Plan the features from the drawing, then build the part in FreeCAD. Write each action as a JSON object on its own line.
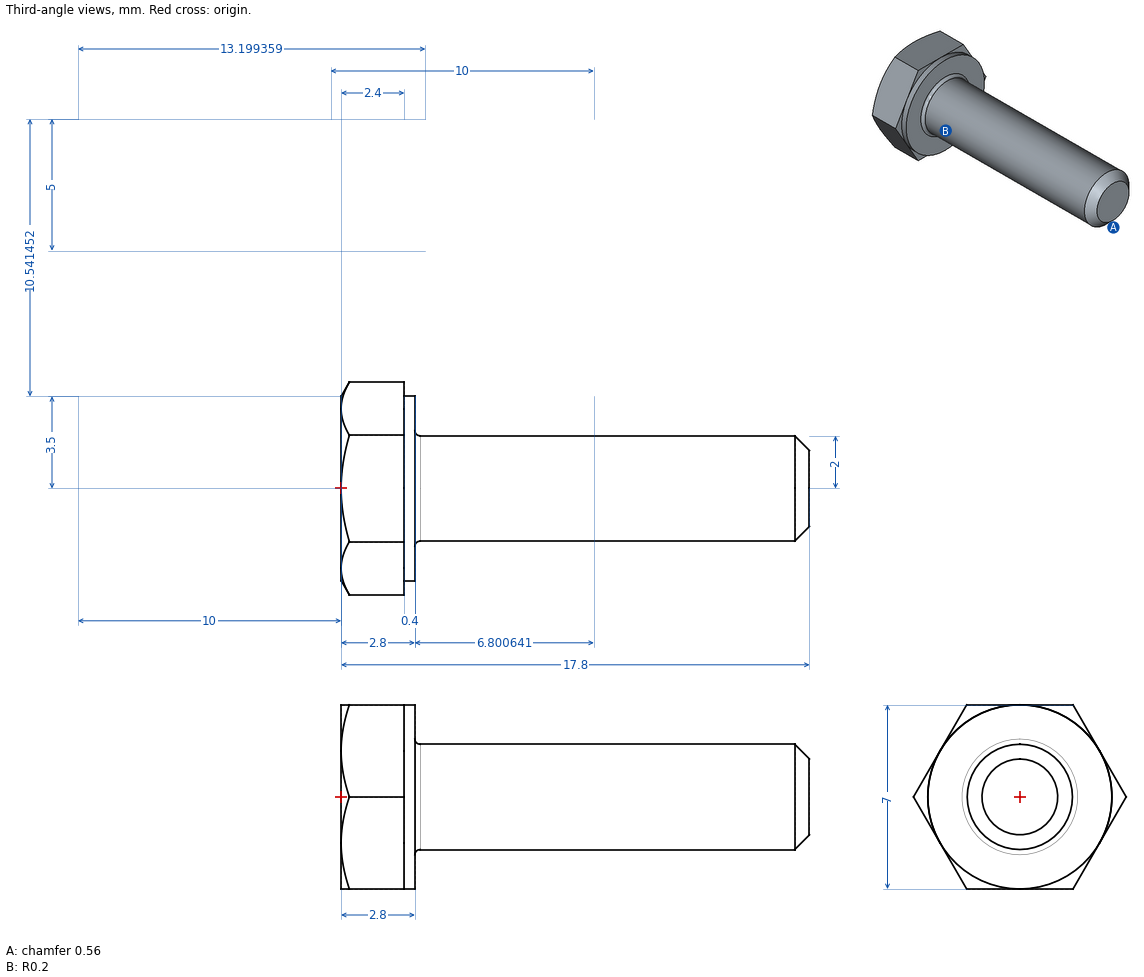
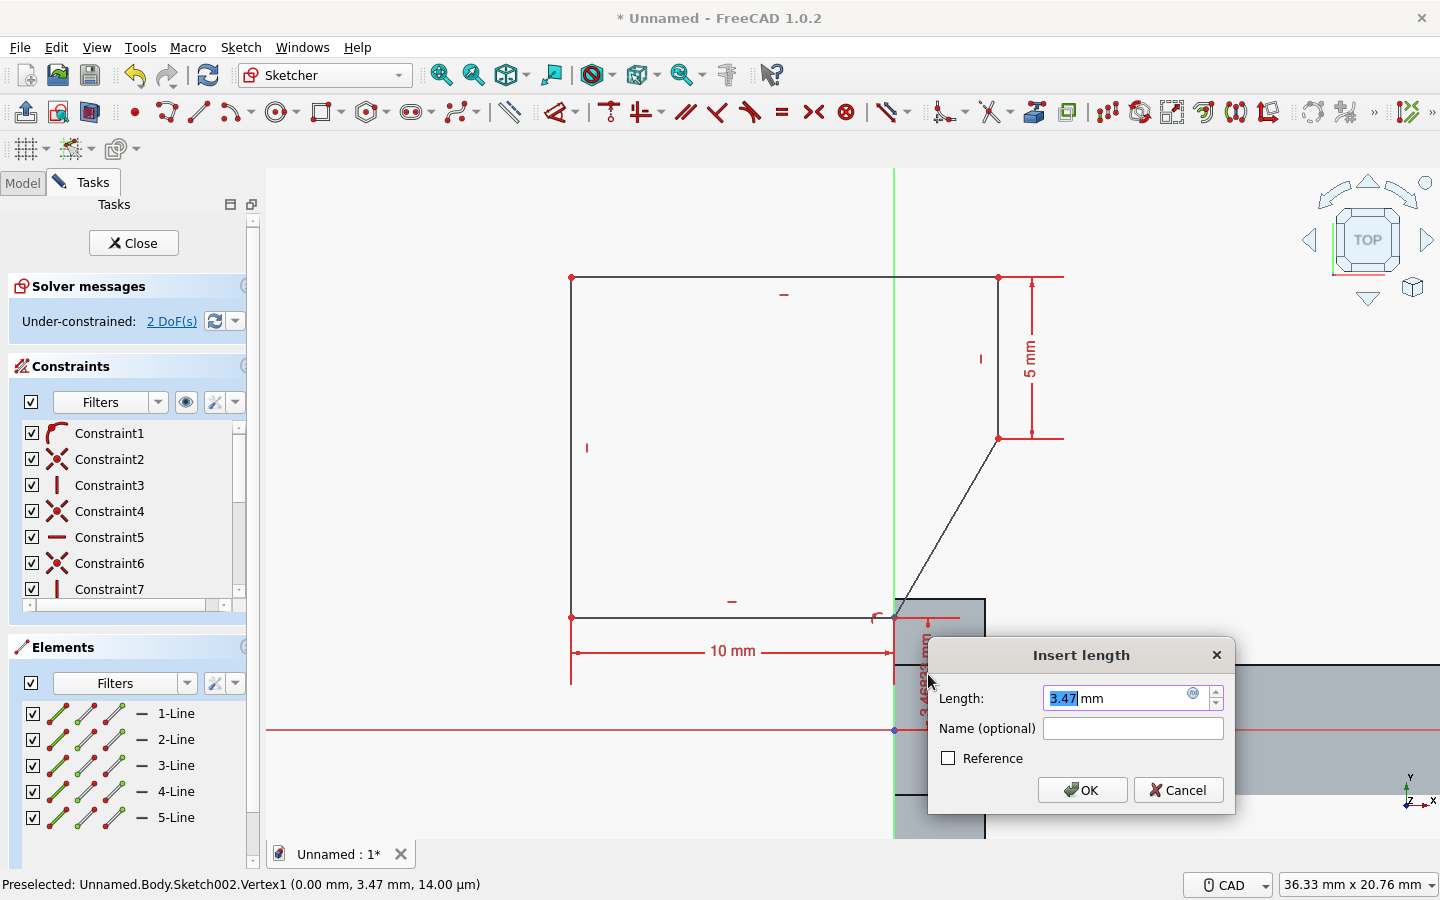
{"action": "type", "text": "3.5"}
{"action": "key", "text": "Return"}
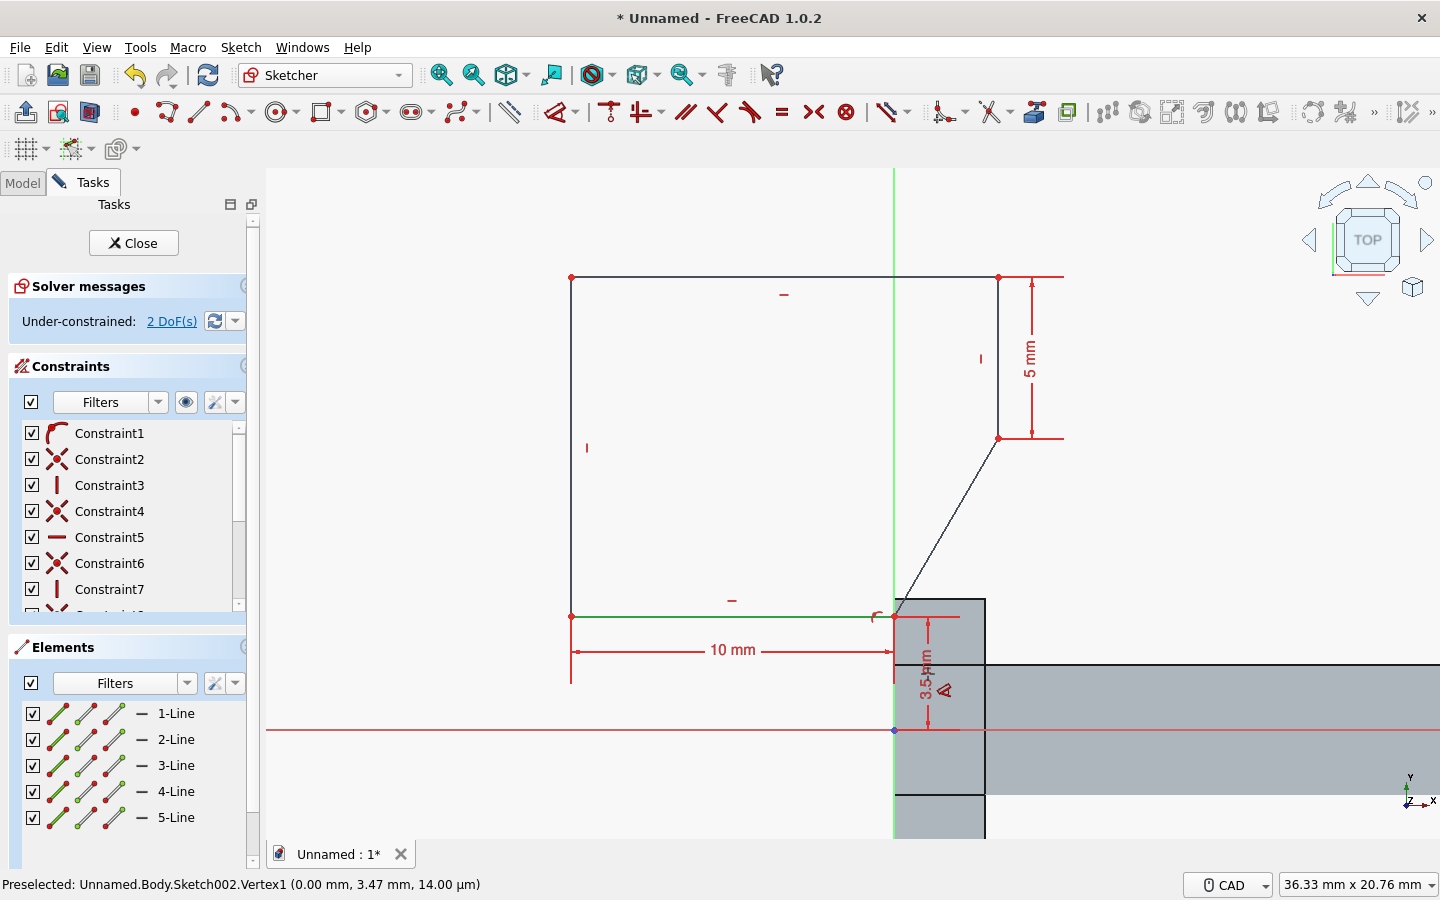
{"action": "left_click", "coordinate": [870, 277]}
{"action": "left_click", "coordinate": [785, 243]}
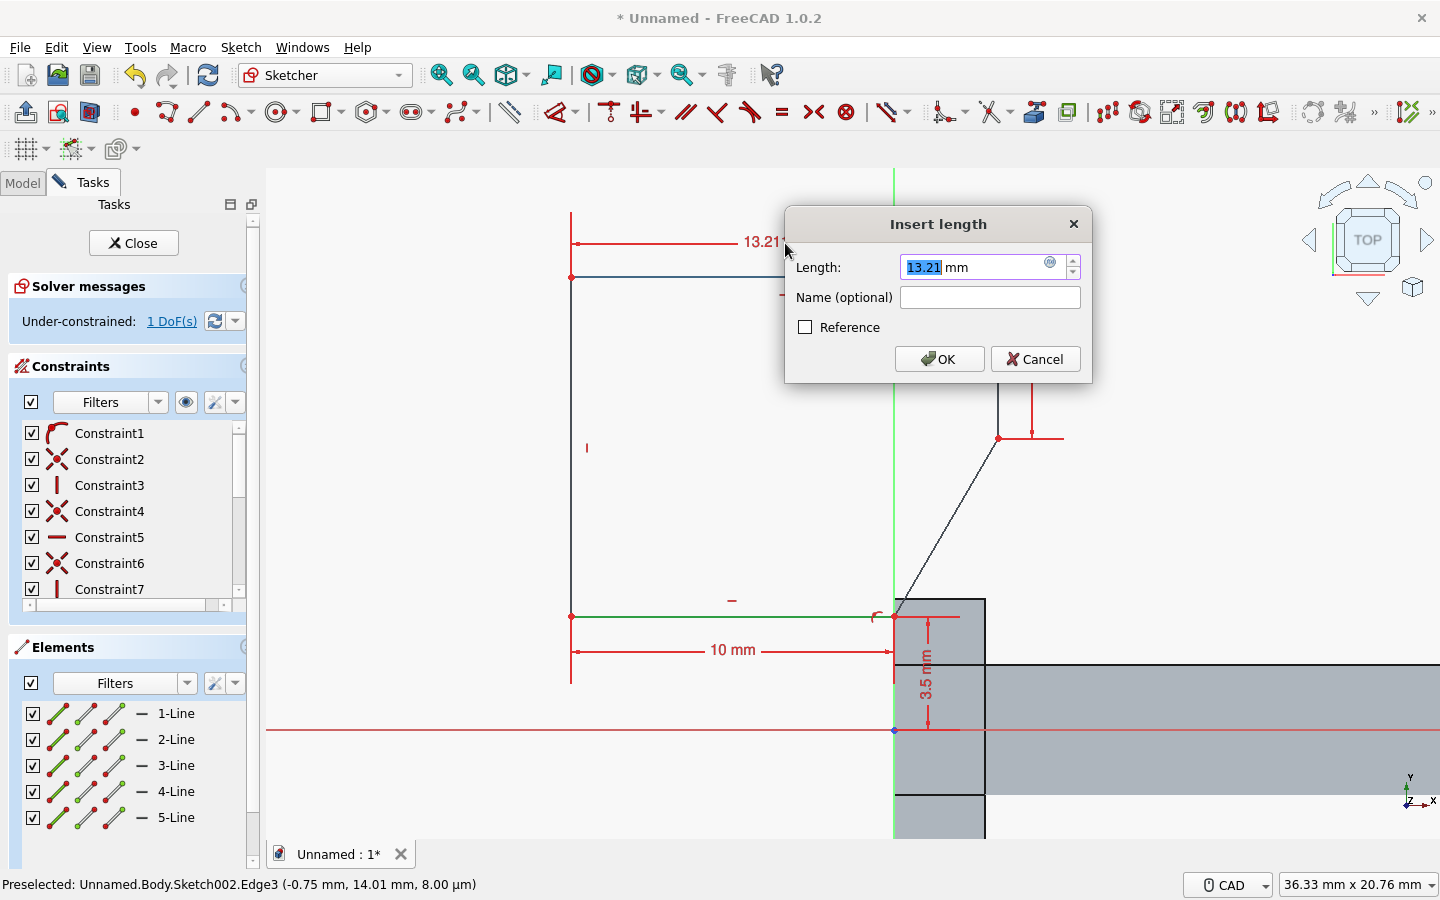
{"action": "type", "text": "13.199359"}
{"action": "key", "text": "Return"}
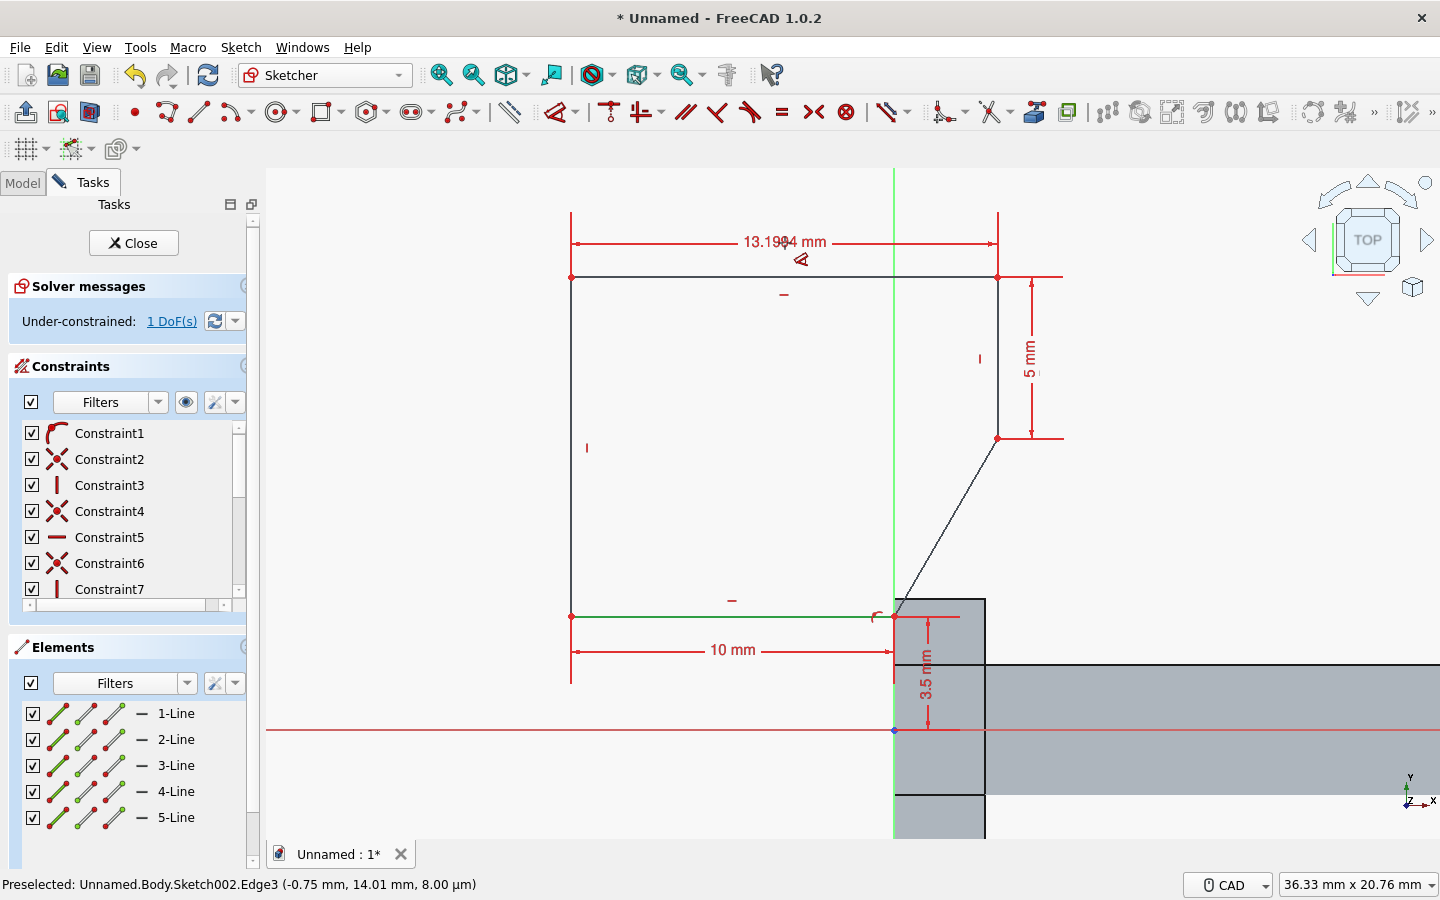
{"action": "left_click", "coordinate": [571, 379]}
{"action": "left_click", "coordinate": [537, 447]}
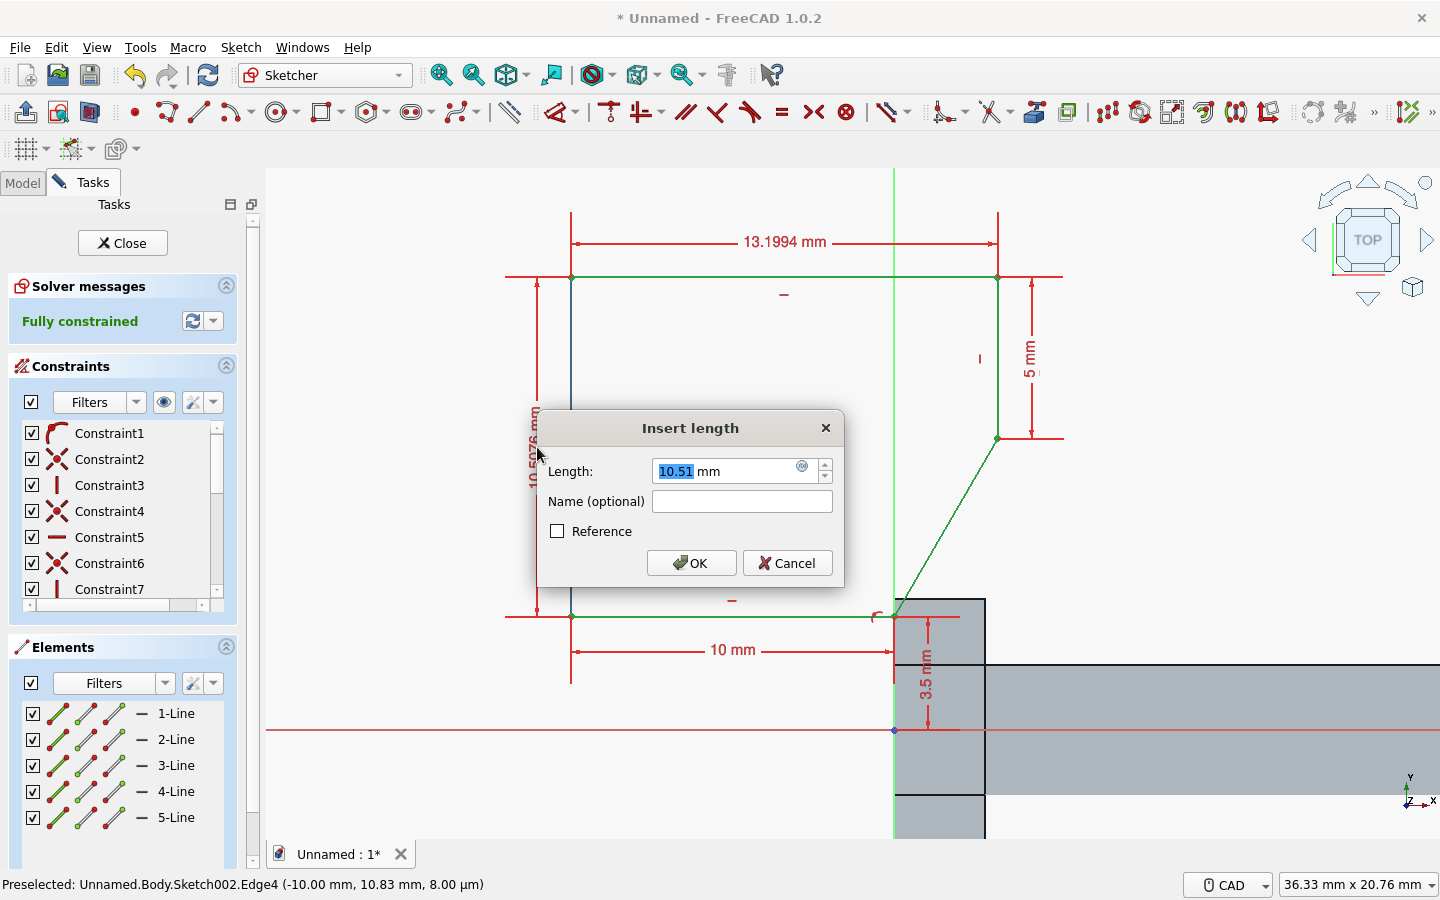
{"action": "type", "text": "10.541452"}
{"action": "key", "text": "Return"}
{"action": "key", "text": "Escape"}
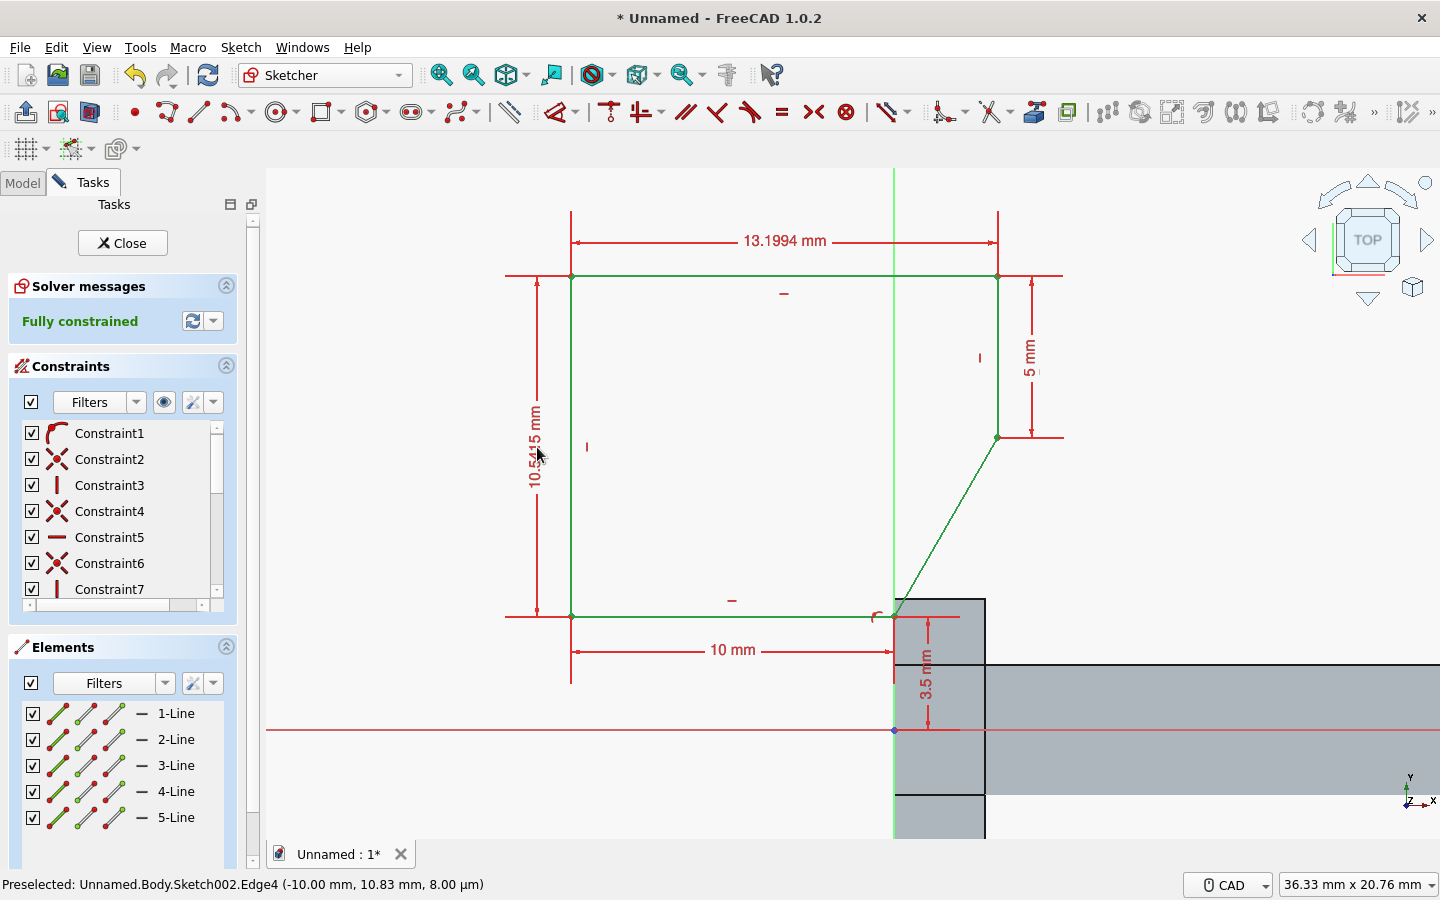
{"action": "left_click", "coordinate": [123, 243]}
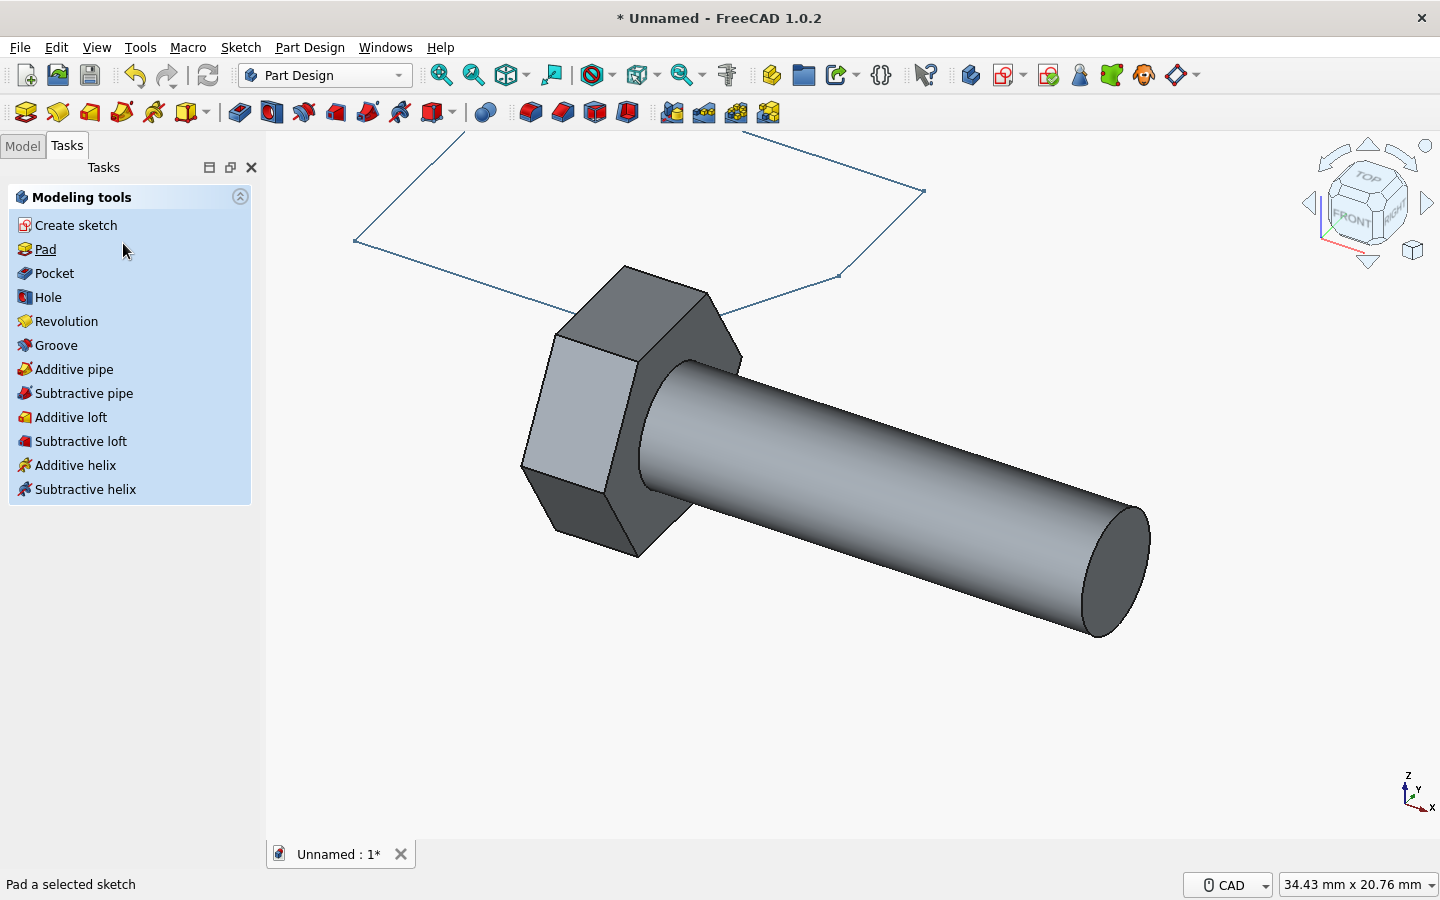
{"action": "left_click", "coordinate": [304, 112]}